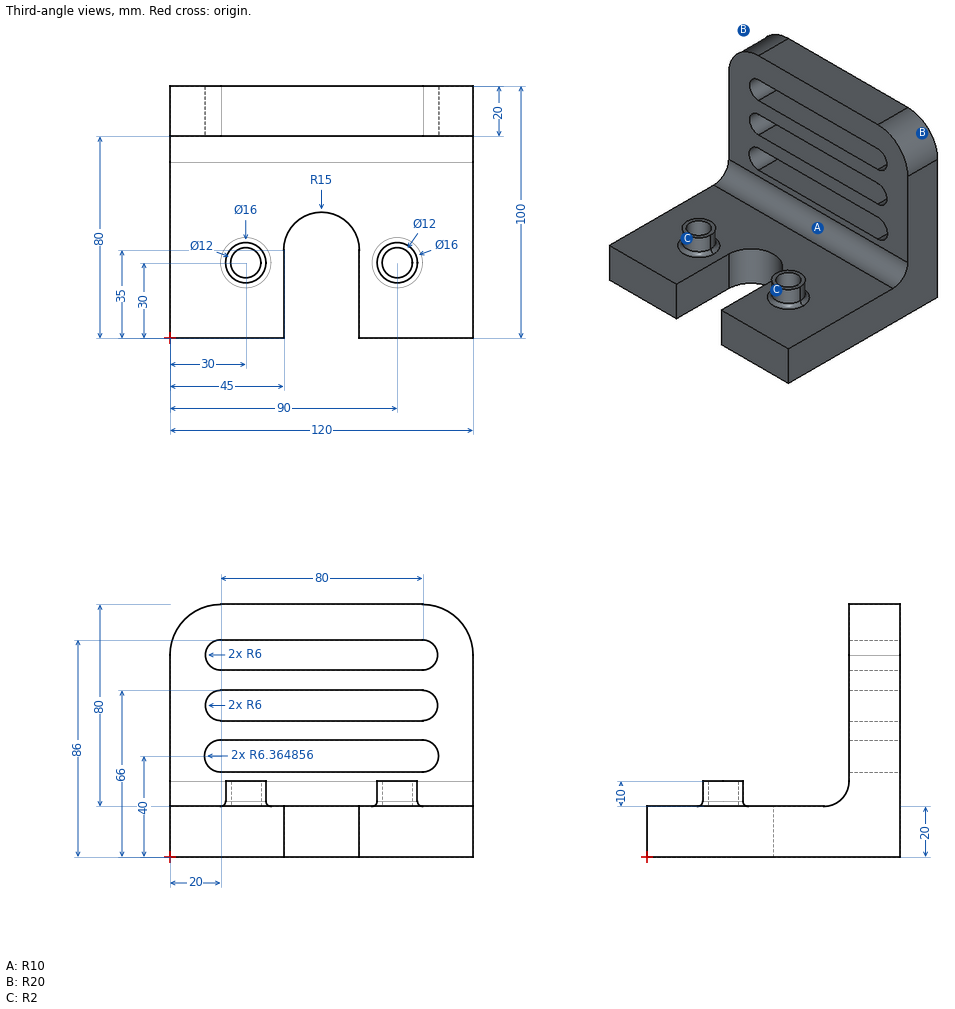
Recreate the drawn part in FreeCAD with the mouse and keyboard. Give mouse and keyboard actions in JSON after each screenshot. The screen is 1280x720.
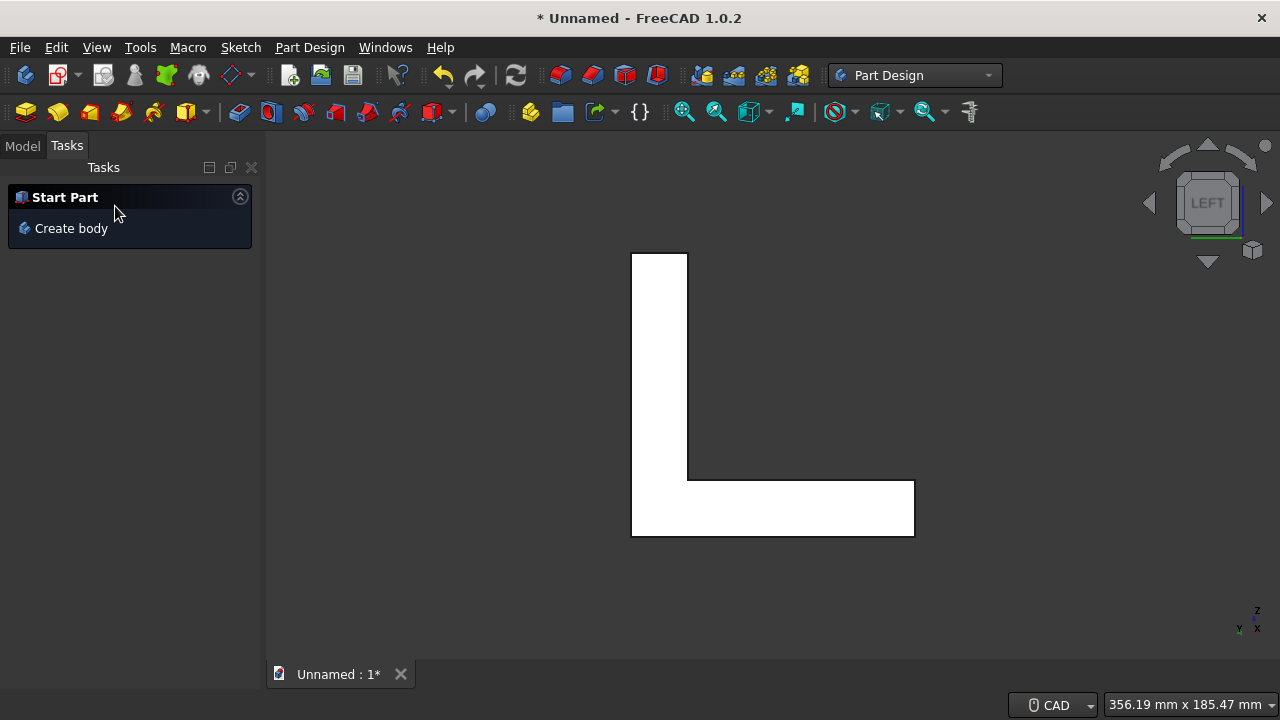
{"action": "key", "text": "v 3"}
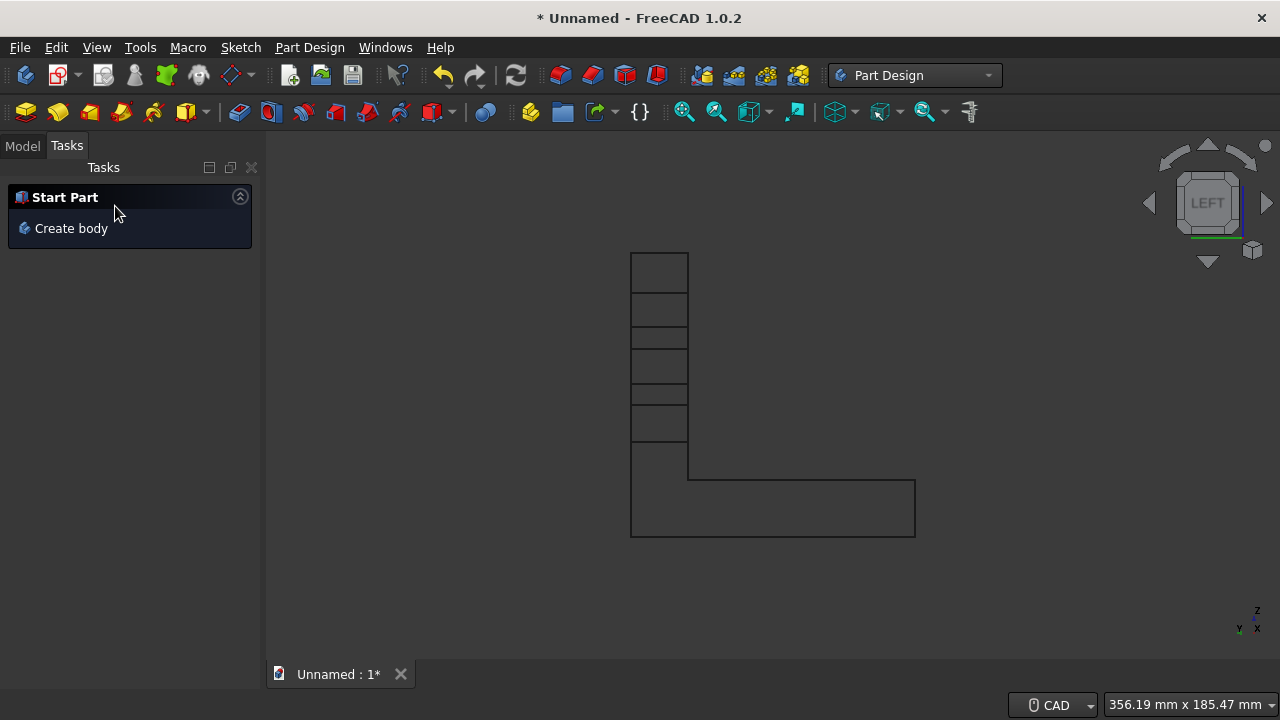
{"action": "key", "text": "0"}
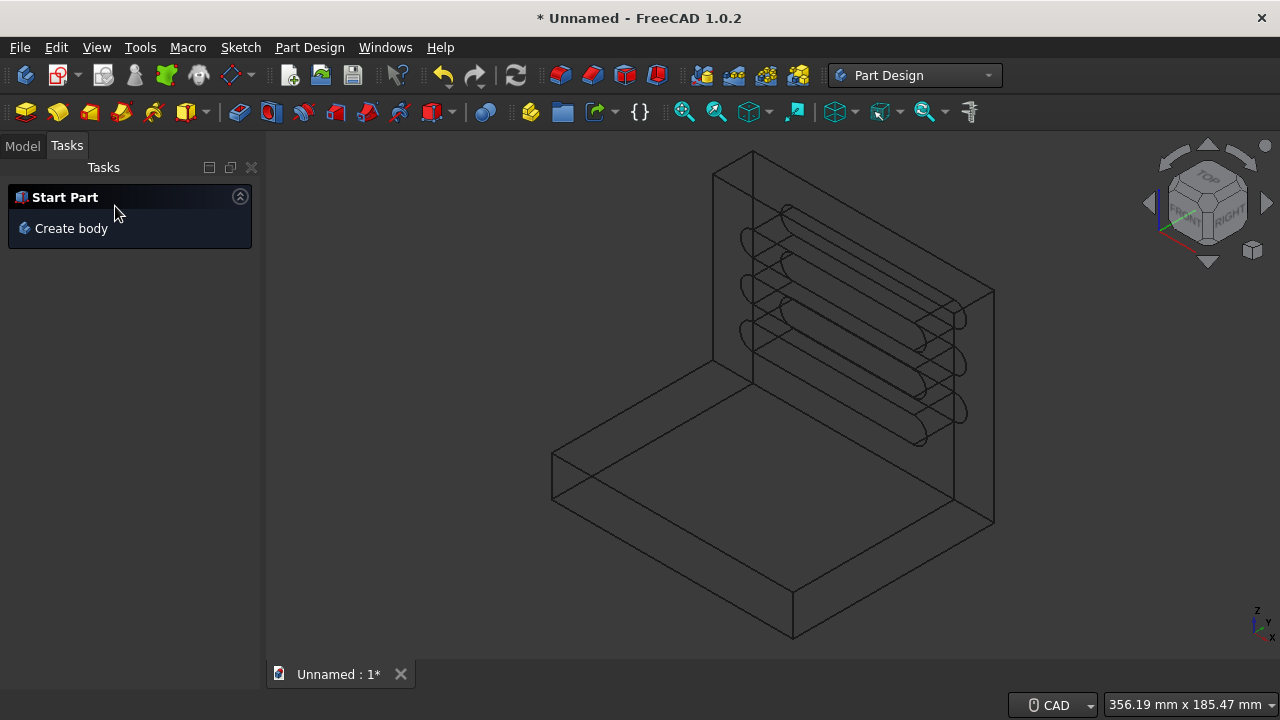
{"action": "left_click", "coordinate": [833, 429]}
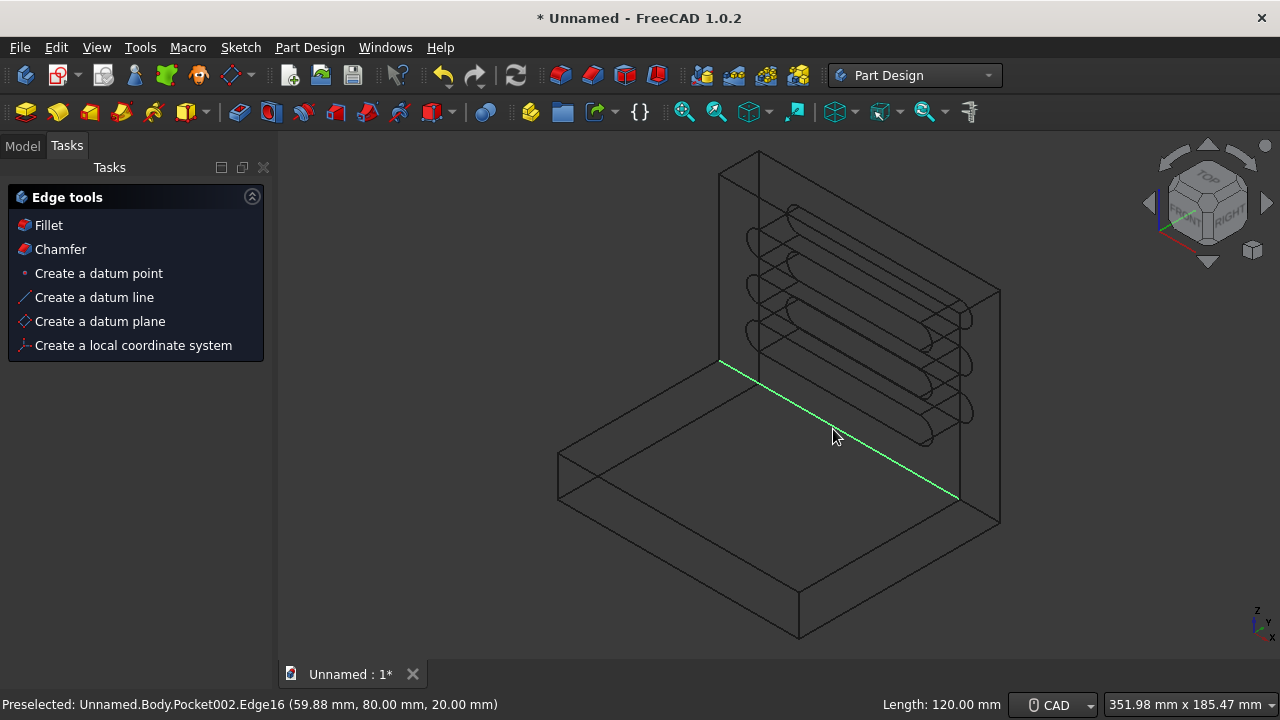
{"action": "key", "text": "v 1"}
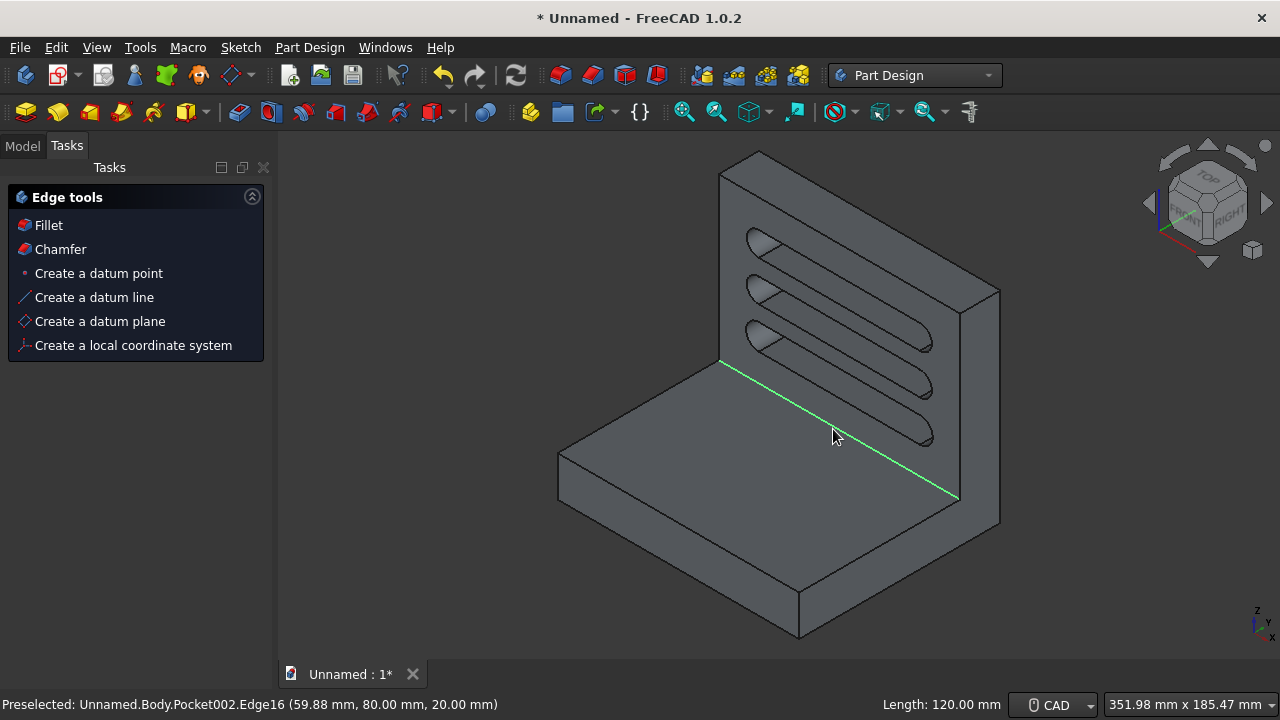
{"action": "left_click", "coordinate": [562, 76]}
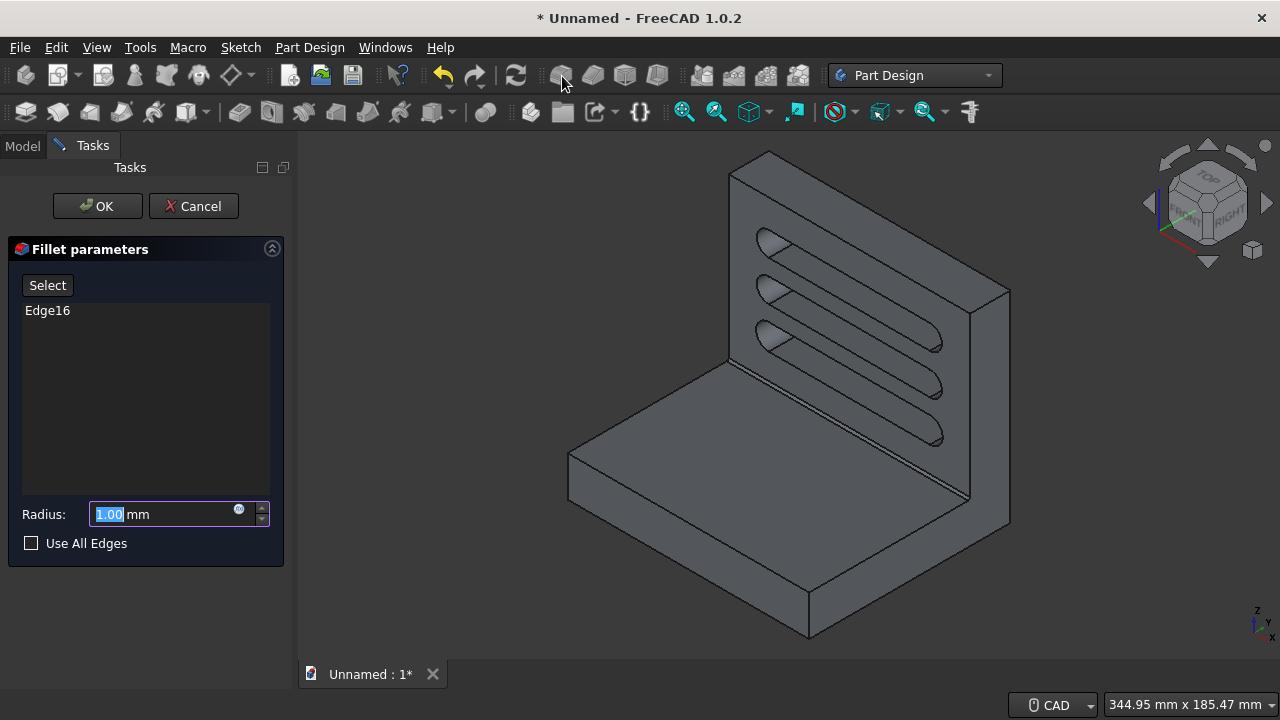
{"action": "type", "text": "10"}
{"action": "key", "text": "Tab"}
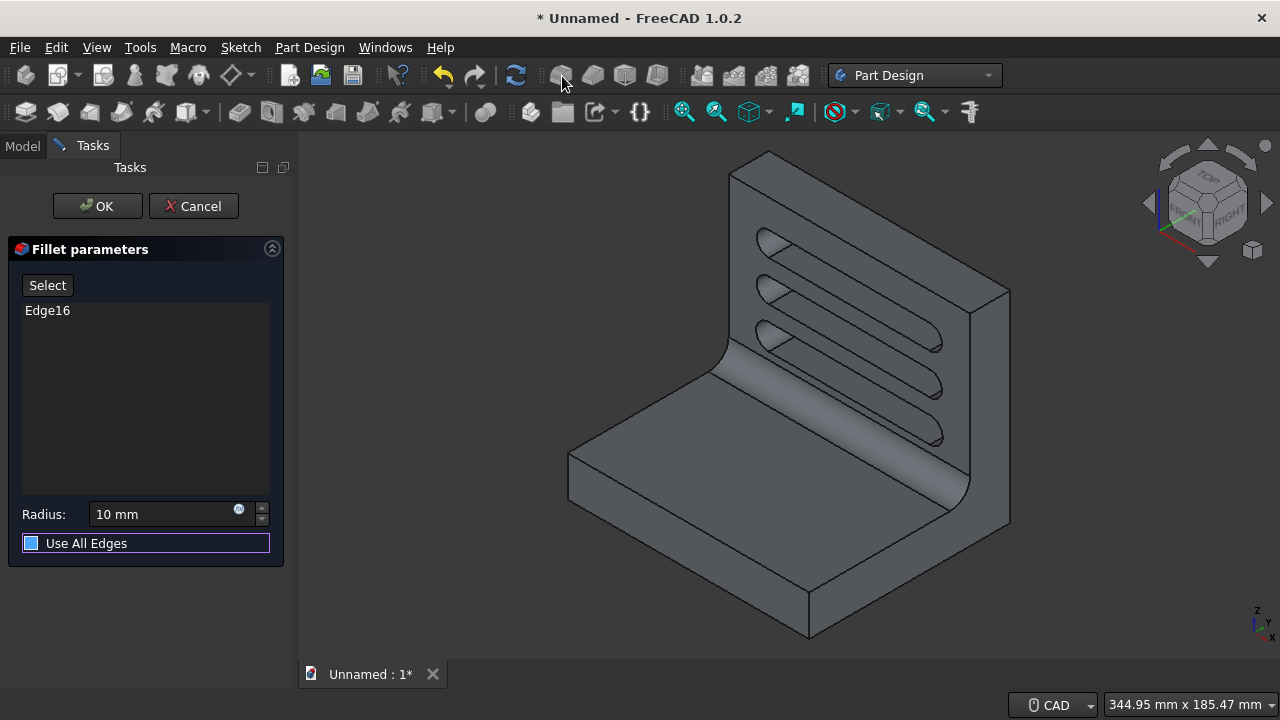
{"action": "left_click", "coordinate": [98, 206]}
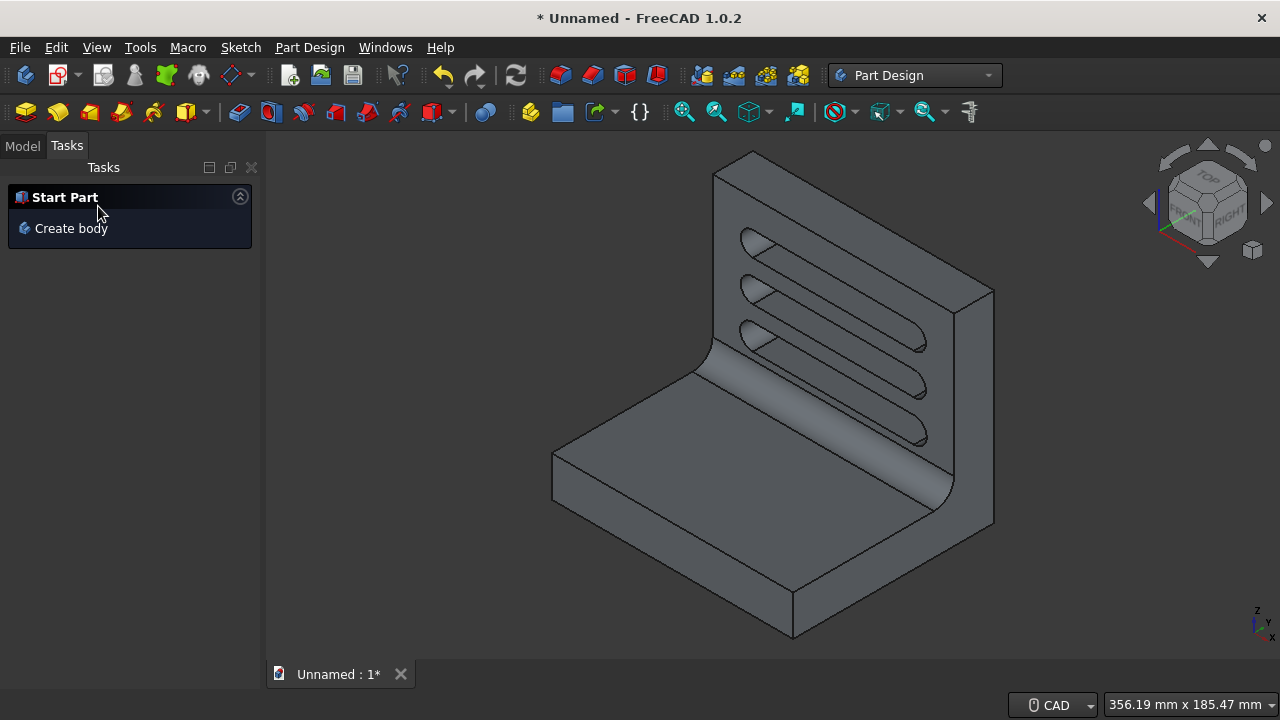
{"action": "left_click", "coordinate": [974, 301]}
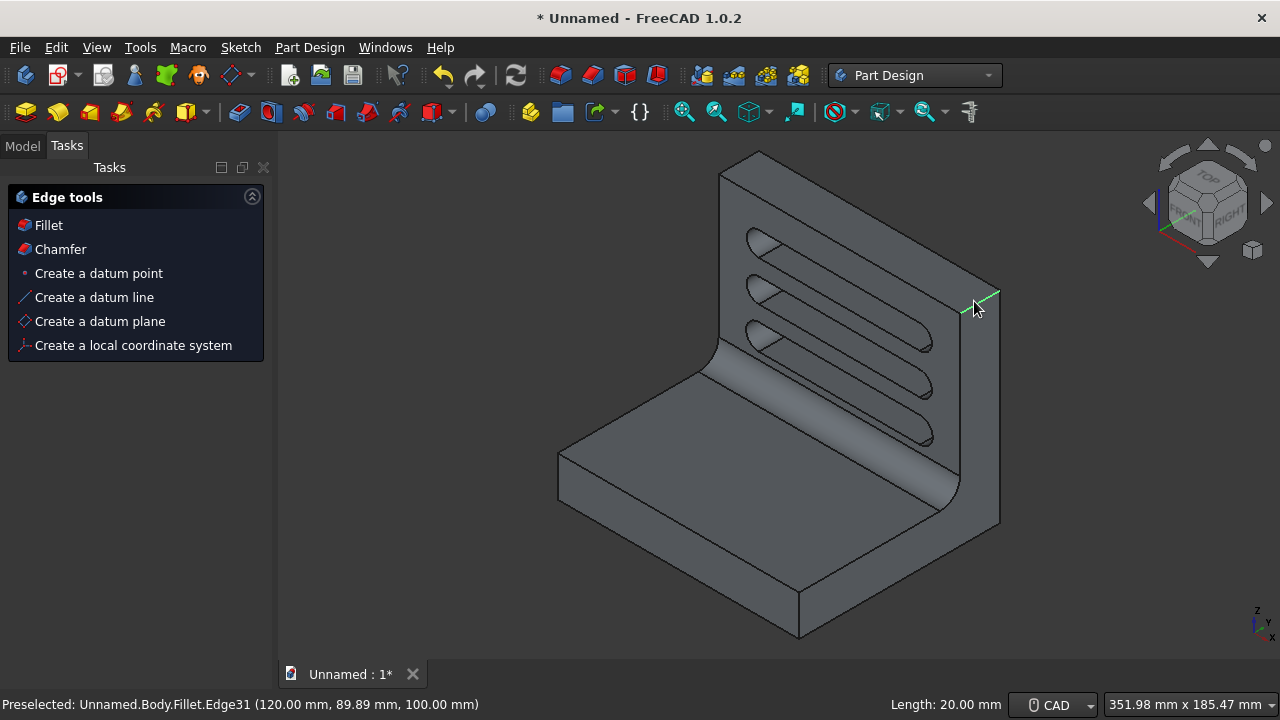
{"action": "key", "text": "2"}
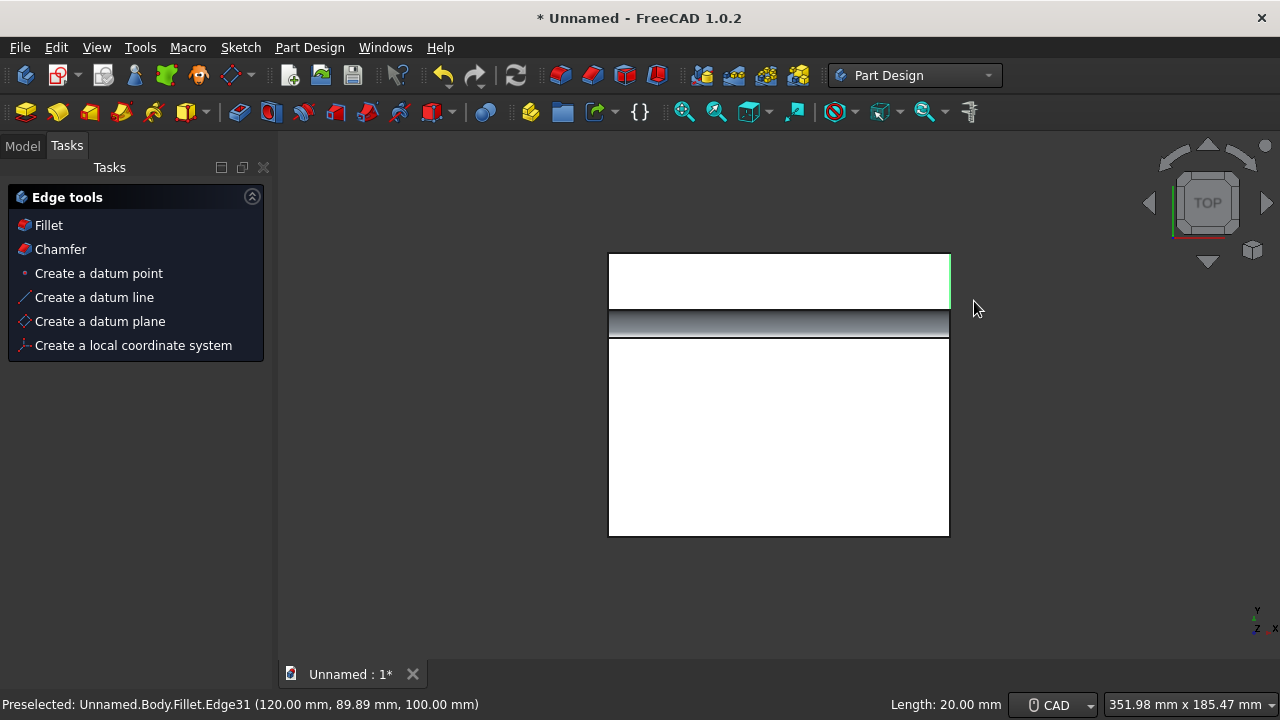
{"action": "left_click", "coordinate": [608, 280], "text": "ctrl"}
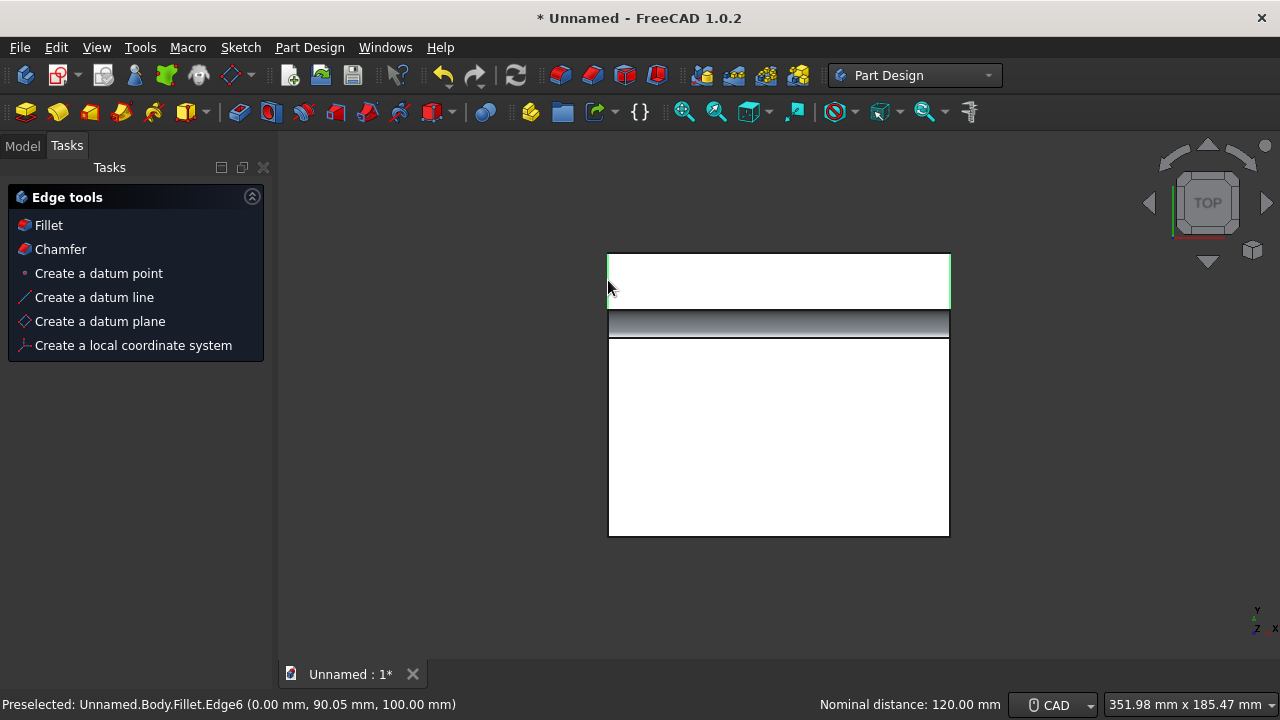
{"action": "left_click", "coordinate": [562, 76]}